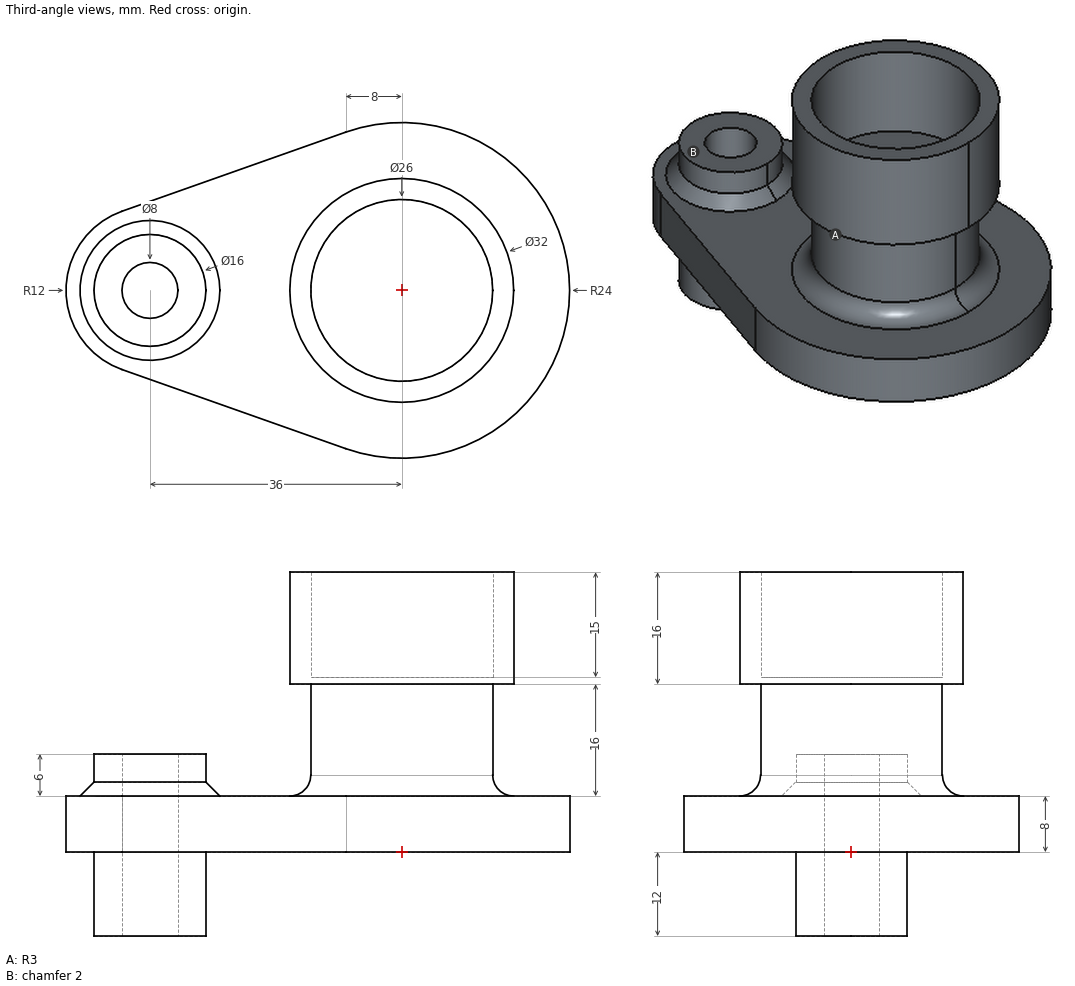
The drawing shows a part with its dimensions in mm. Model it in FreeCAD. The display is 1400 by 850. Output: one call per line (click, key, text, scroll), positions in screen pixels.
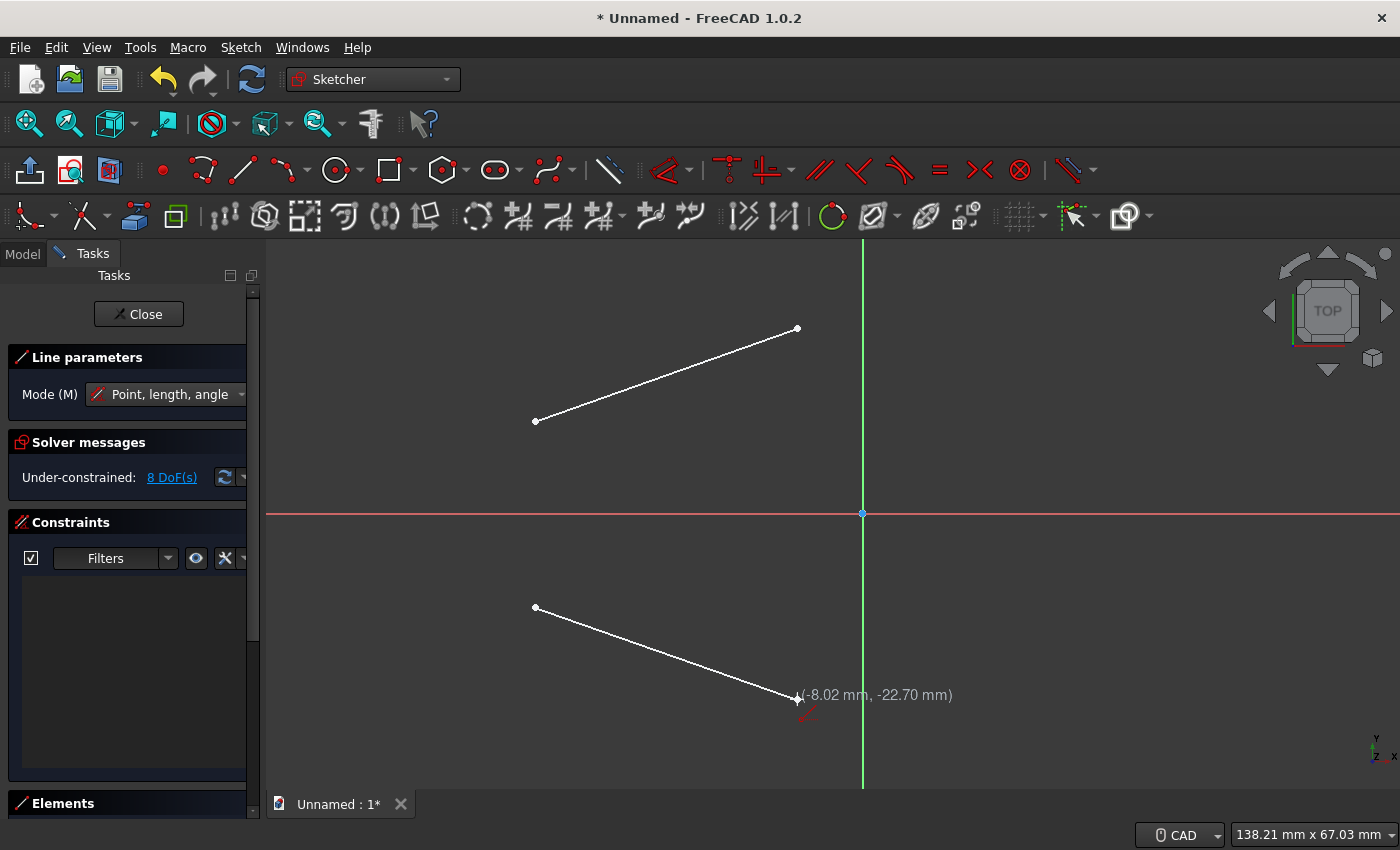
key(g)
key(3)
key(a)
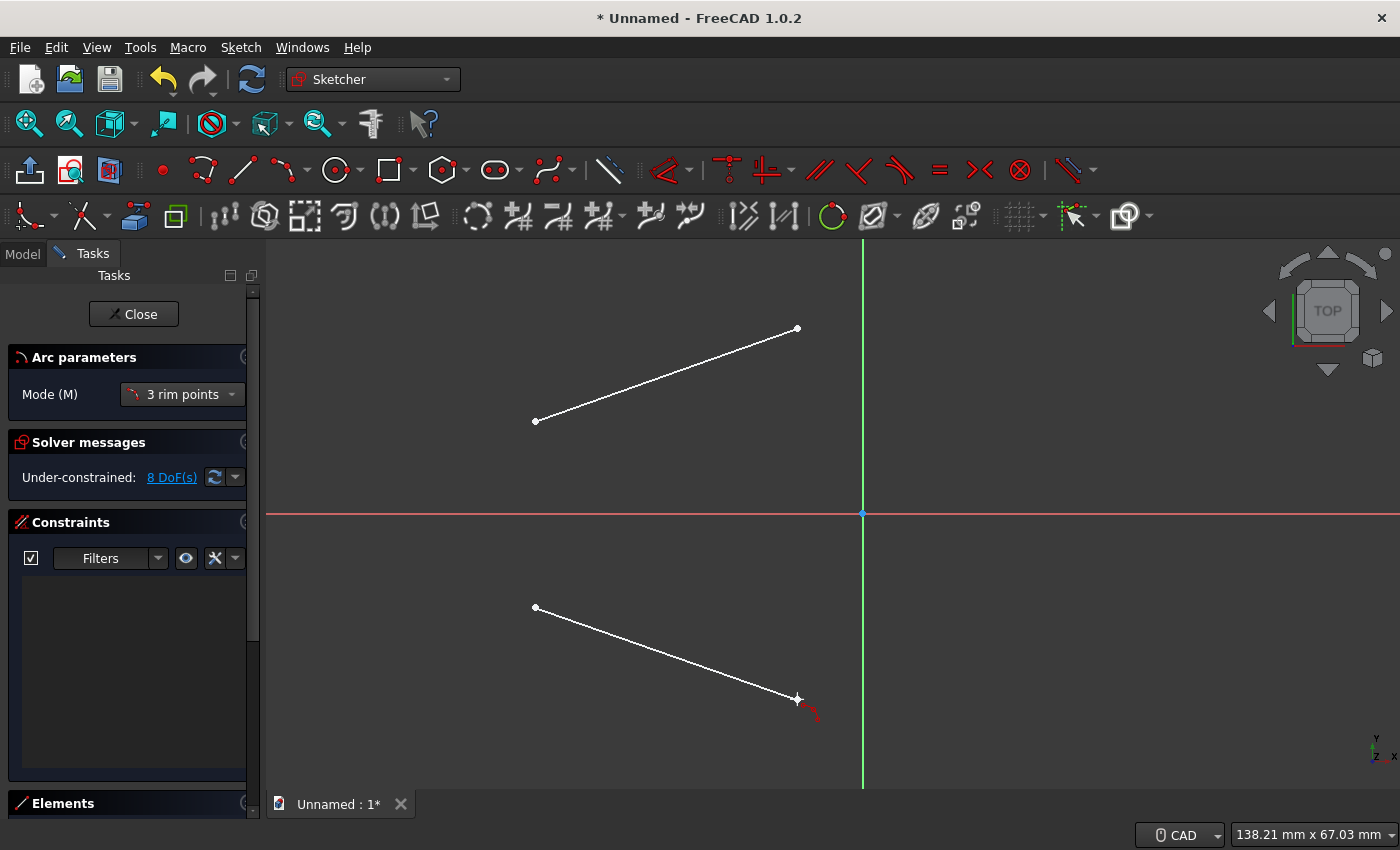
click(535, 422)
click(535, 608)
click(472, 490)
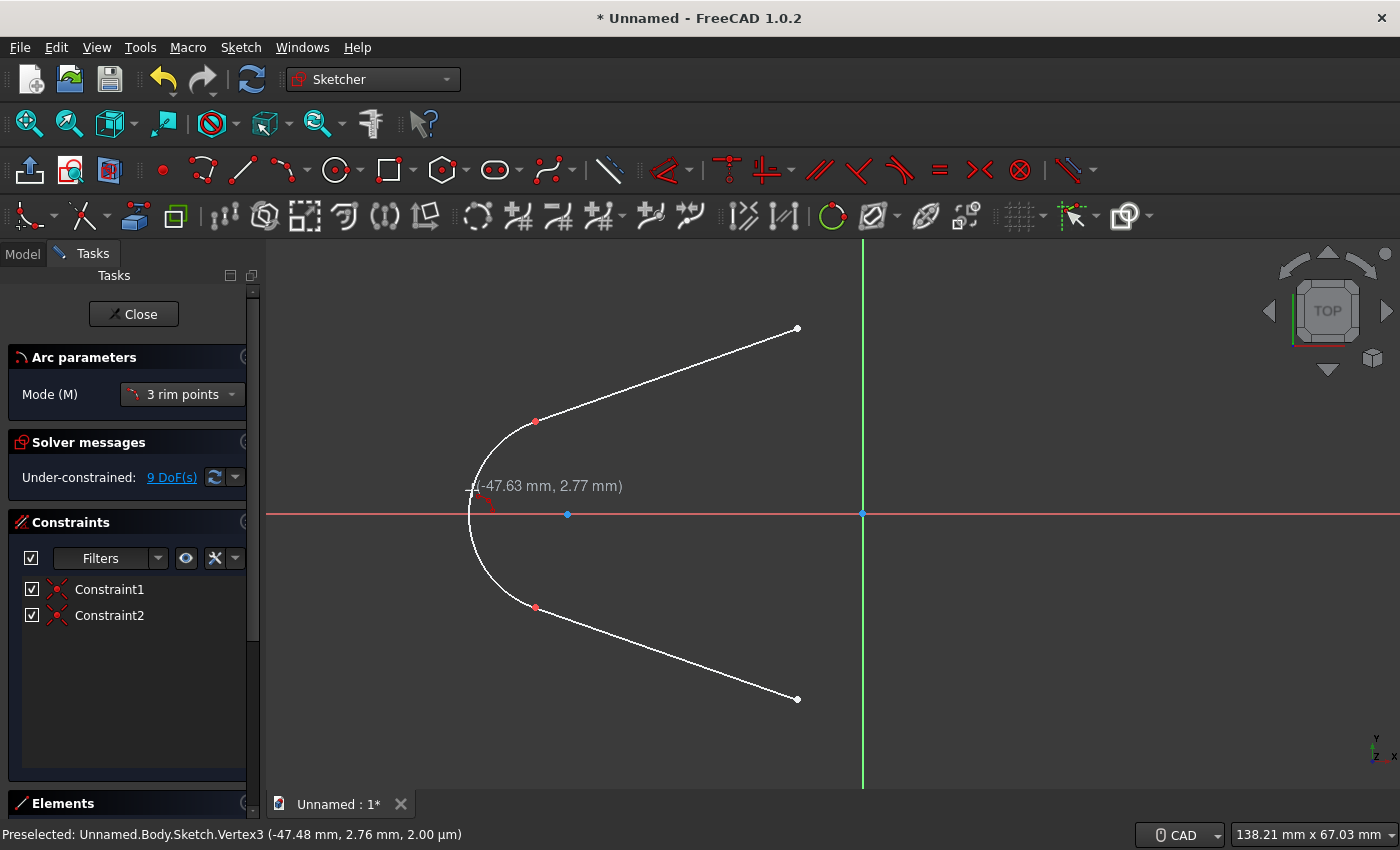
click(797, 700)
click(797, 329)
click(1045, 587)
key(Escape)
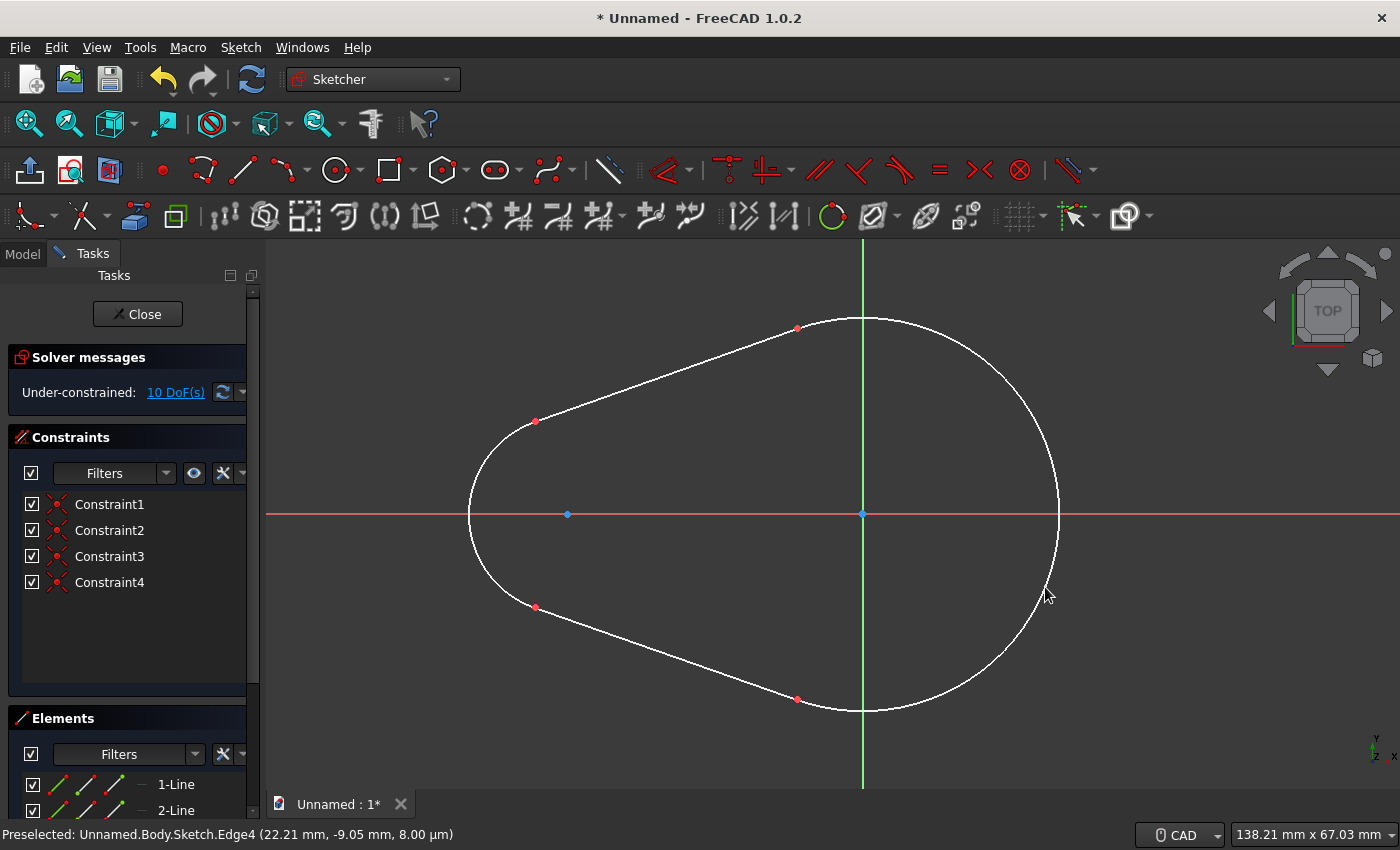
click(718, 357)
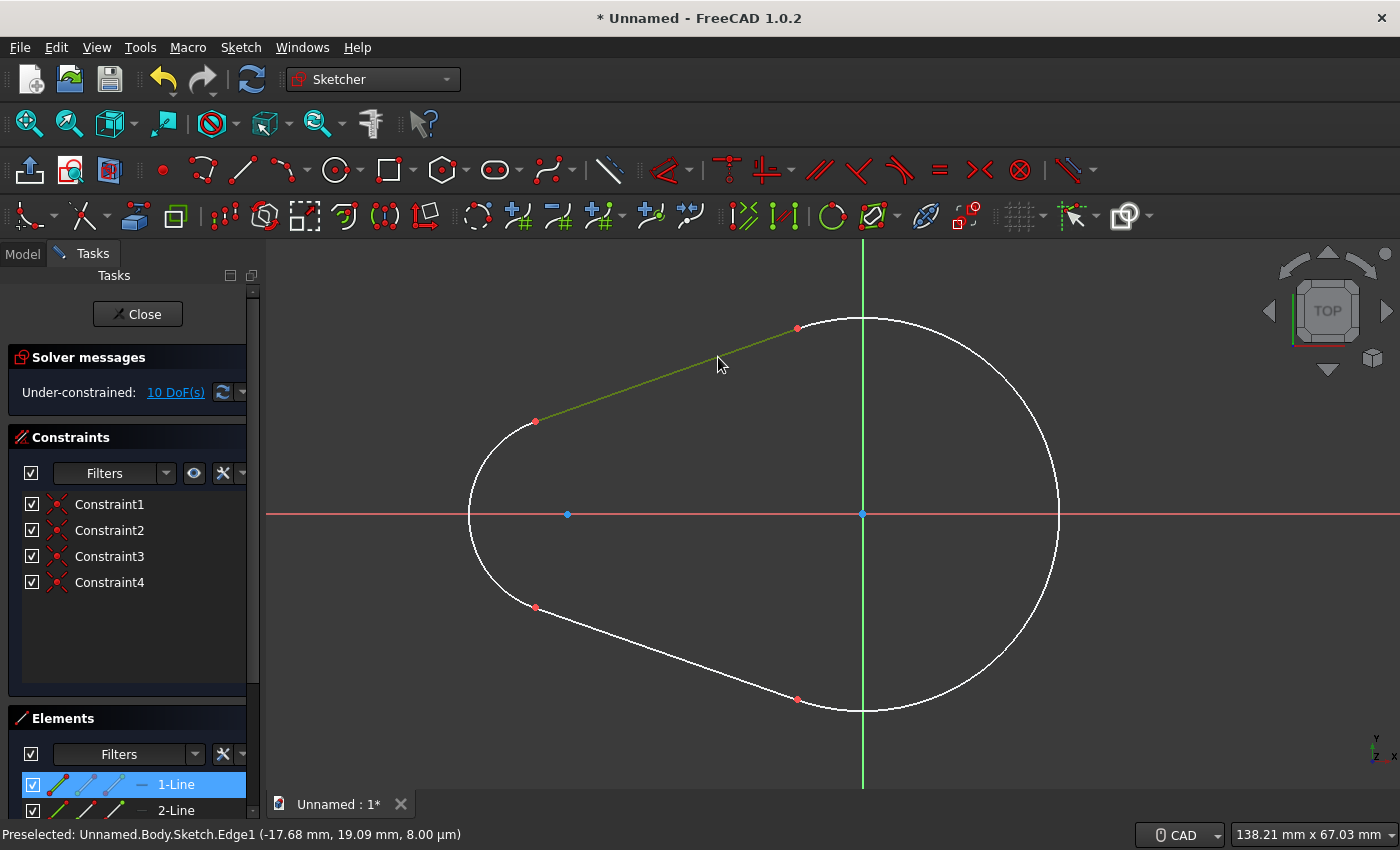
click(481, 468)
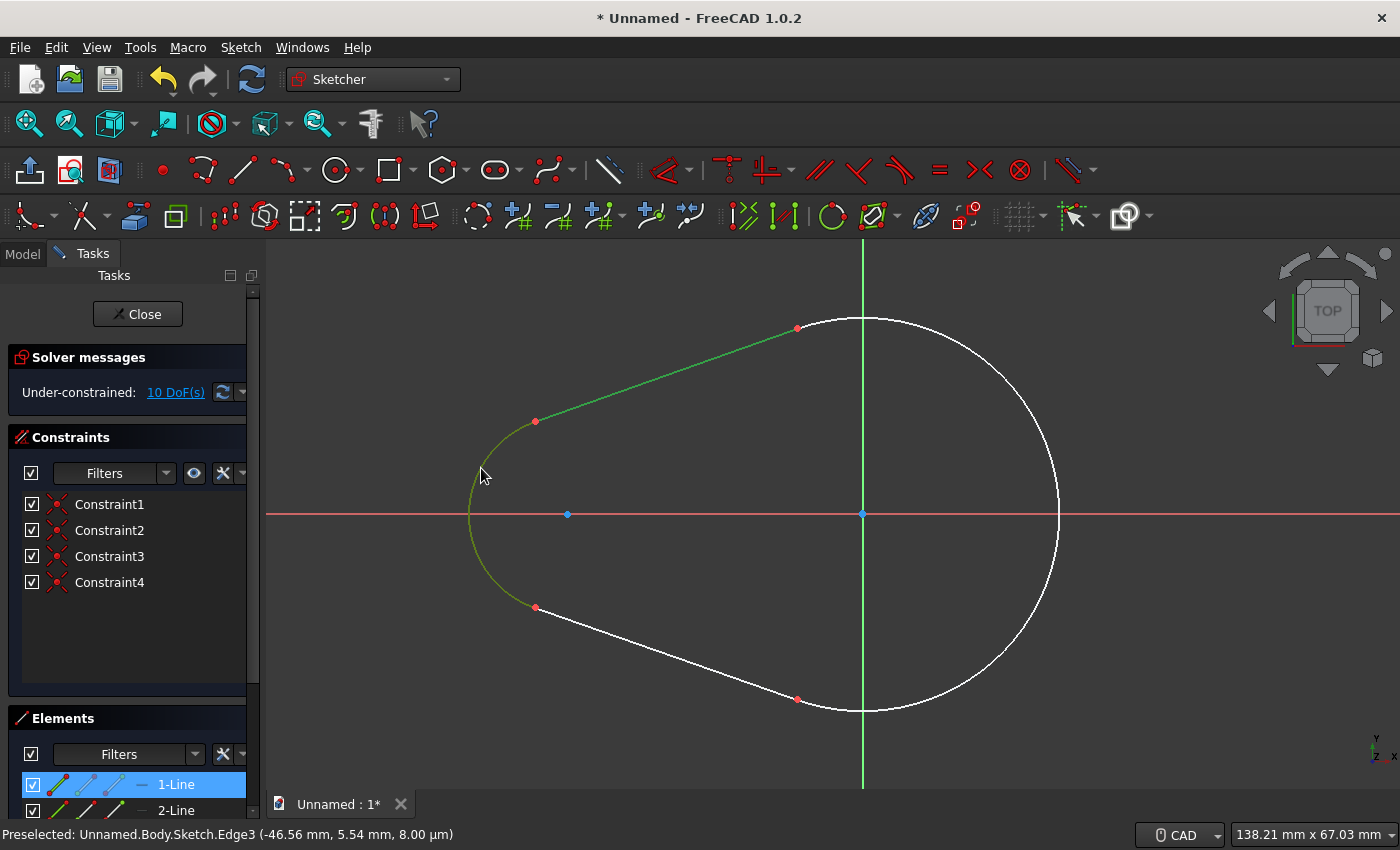
key(t)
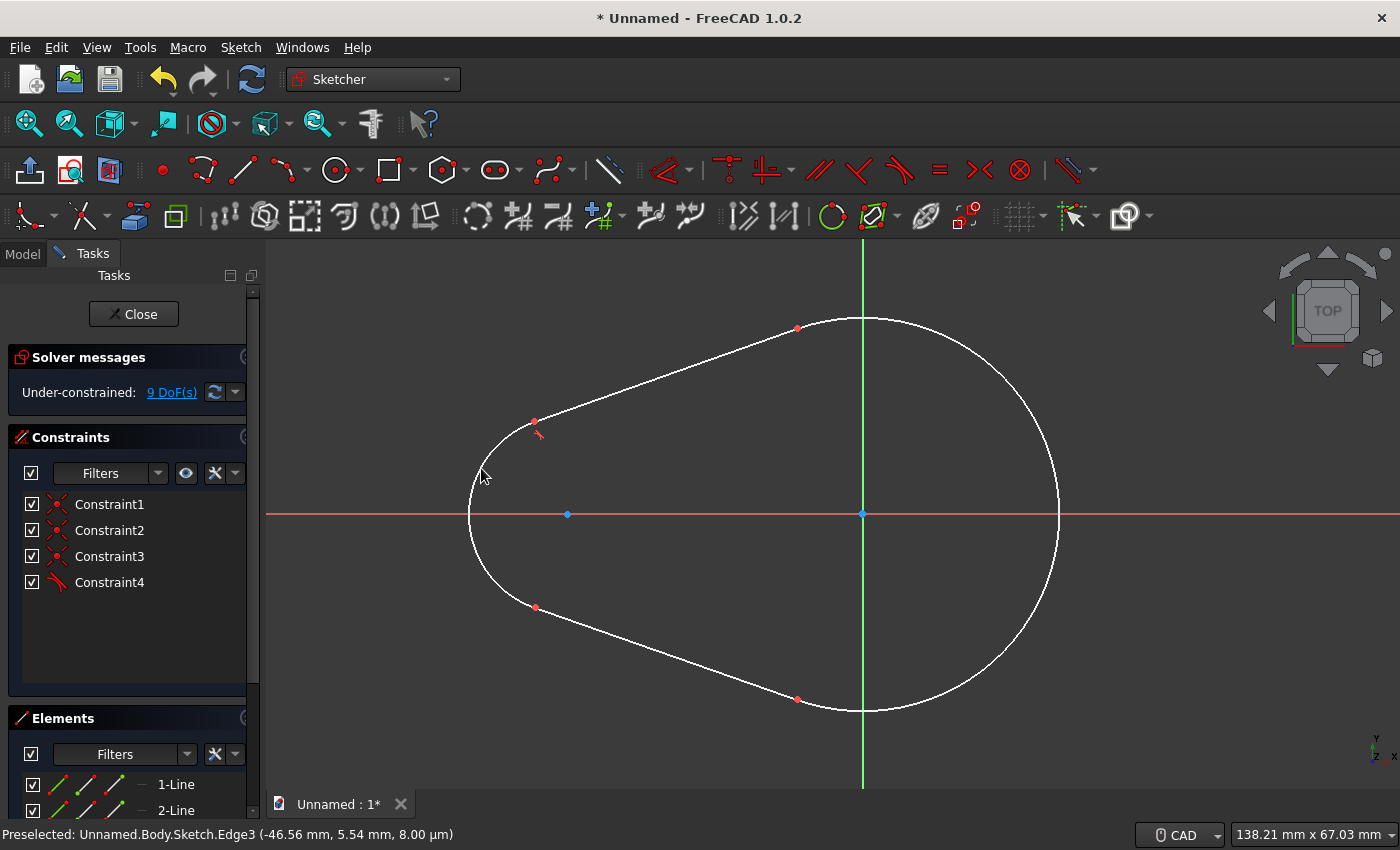
click(718, 357)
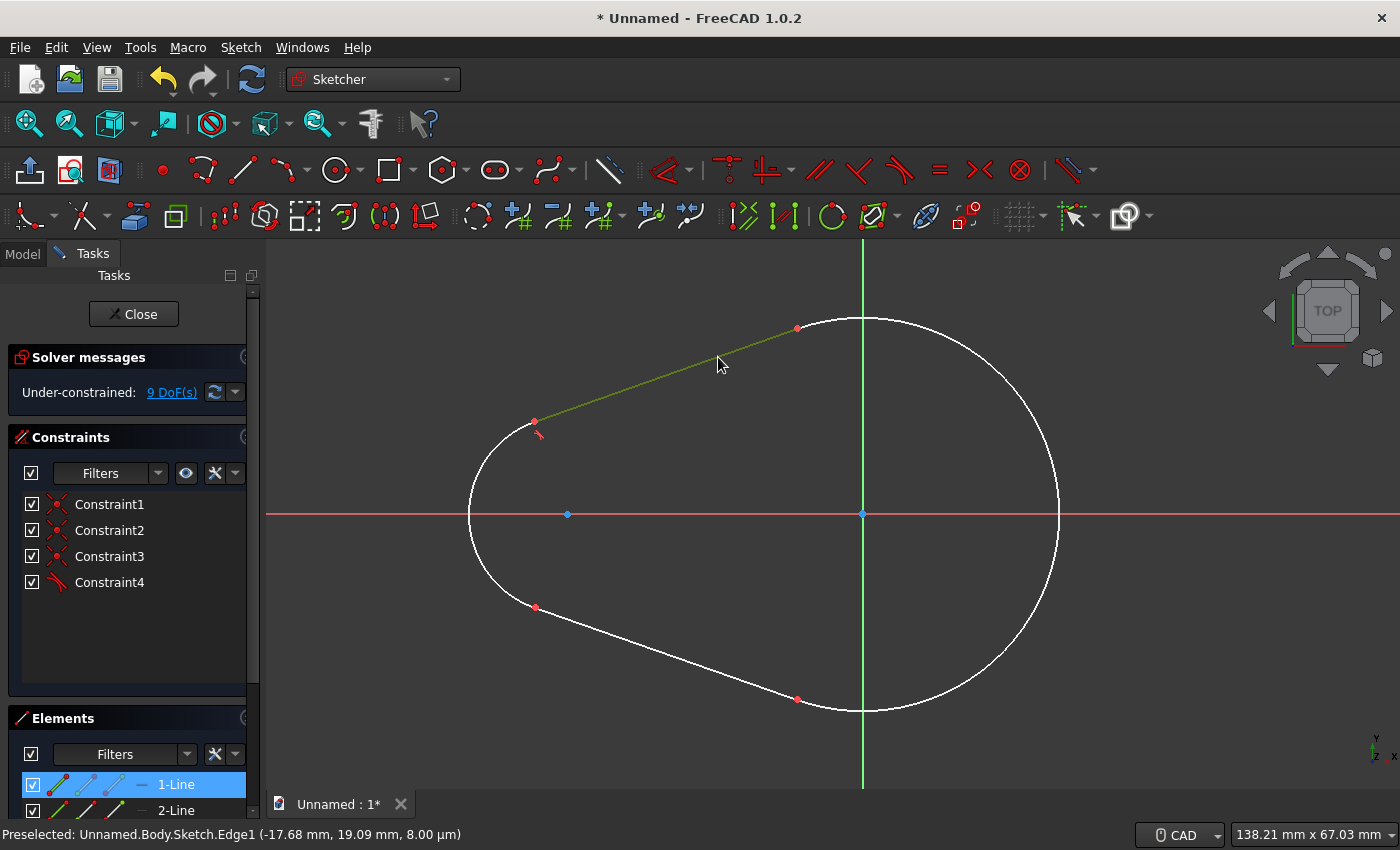
click(1005, 651)